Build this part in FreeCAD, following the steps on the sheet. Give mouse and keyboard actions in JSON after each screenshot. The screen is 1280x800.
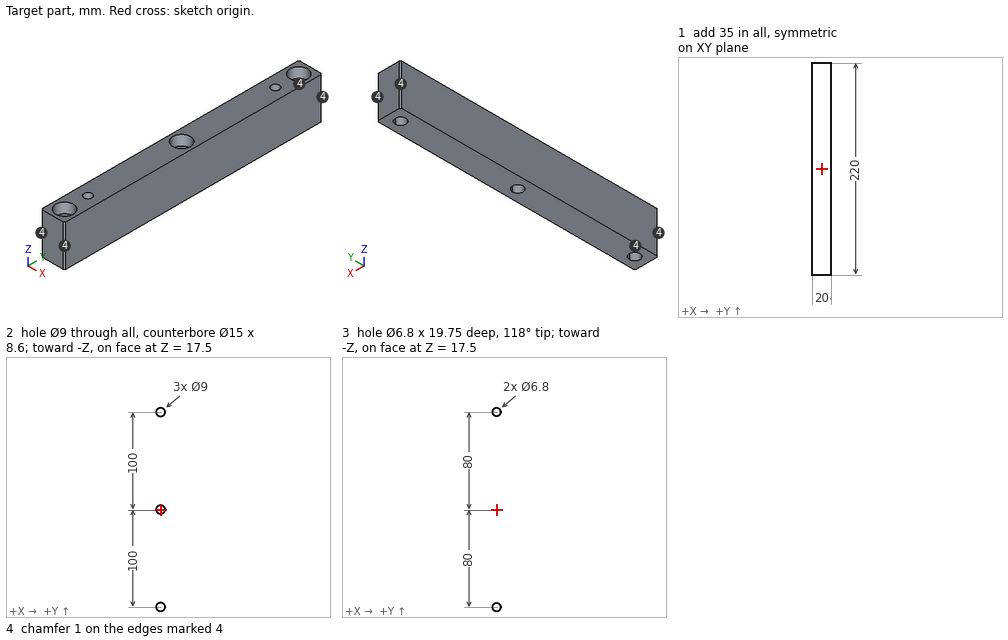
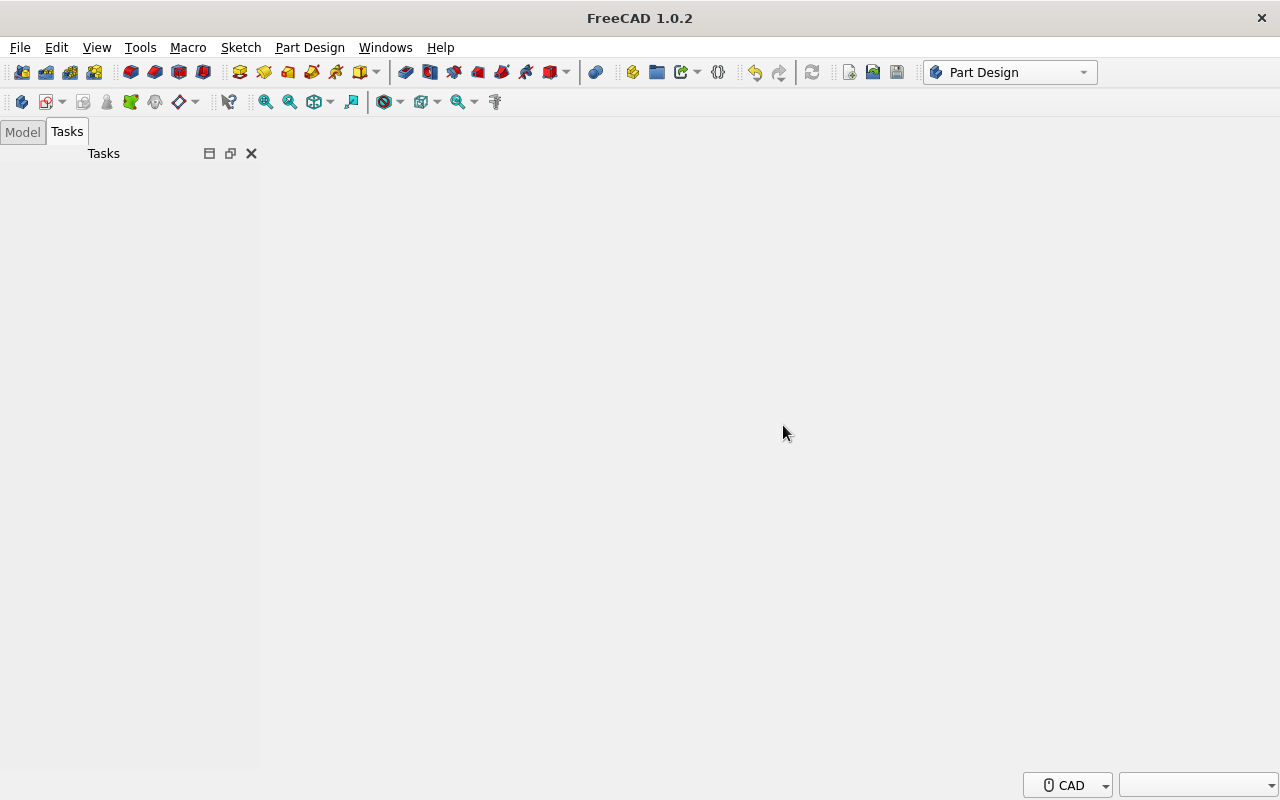
{"action": "left_click", "coordinate": [850, 72]}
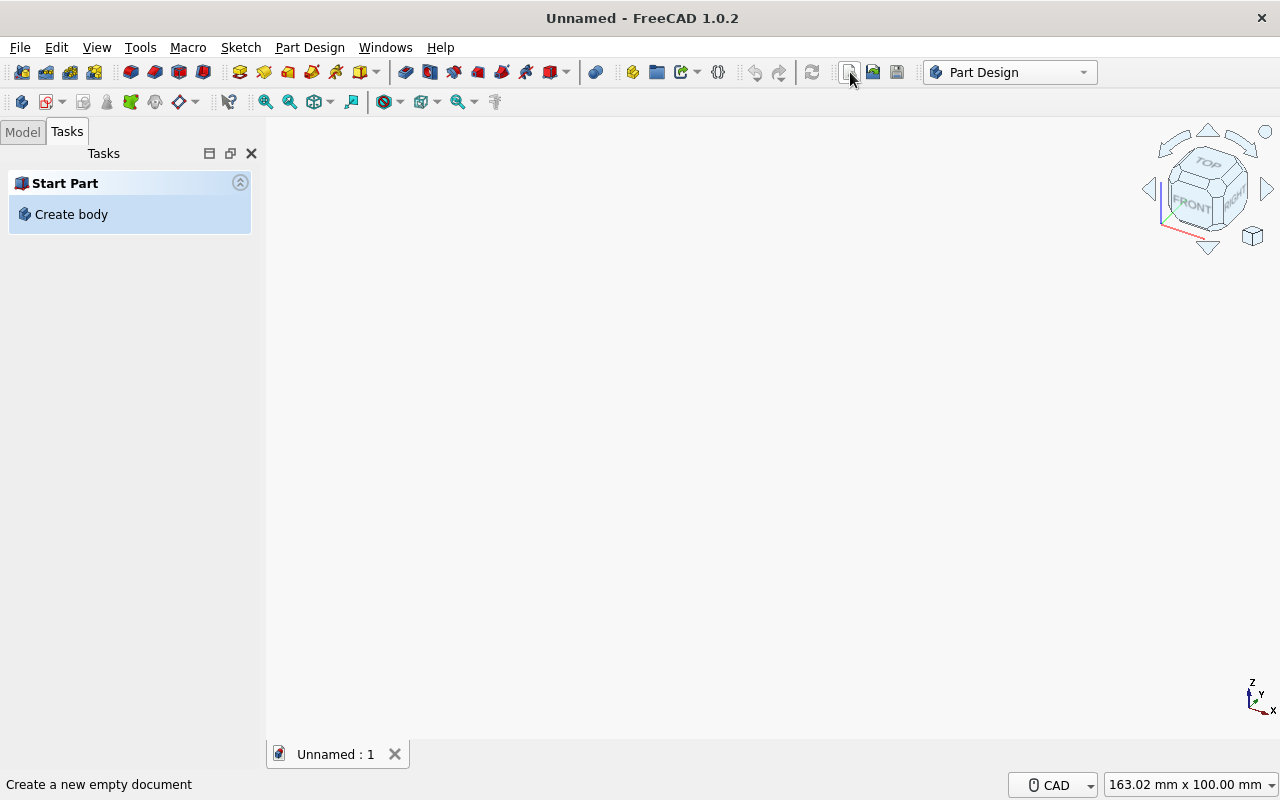
{"action": "left_click", "coordinate": [46, 102]}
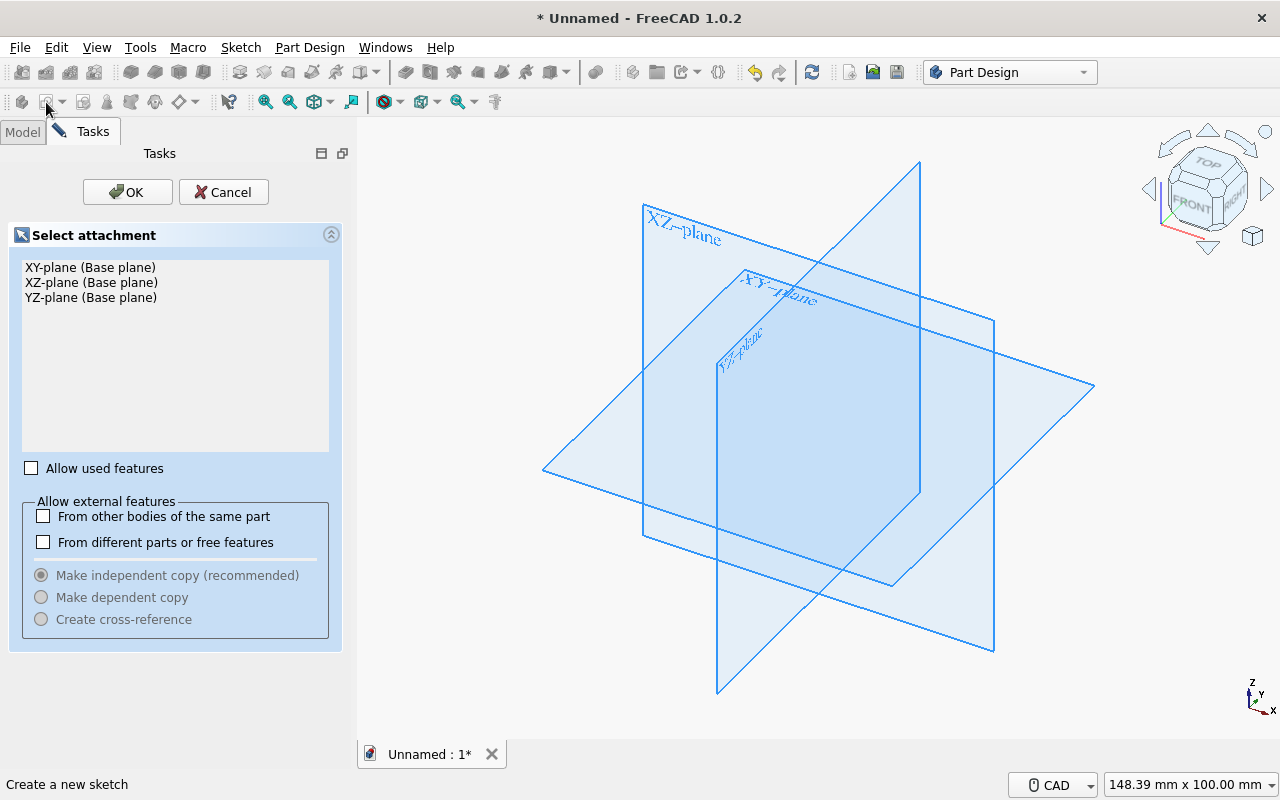
{"action": "left_click", "coordinate": [82, 268]}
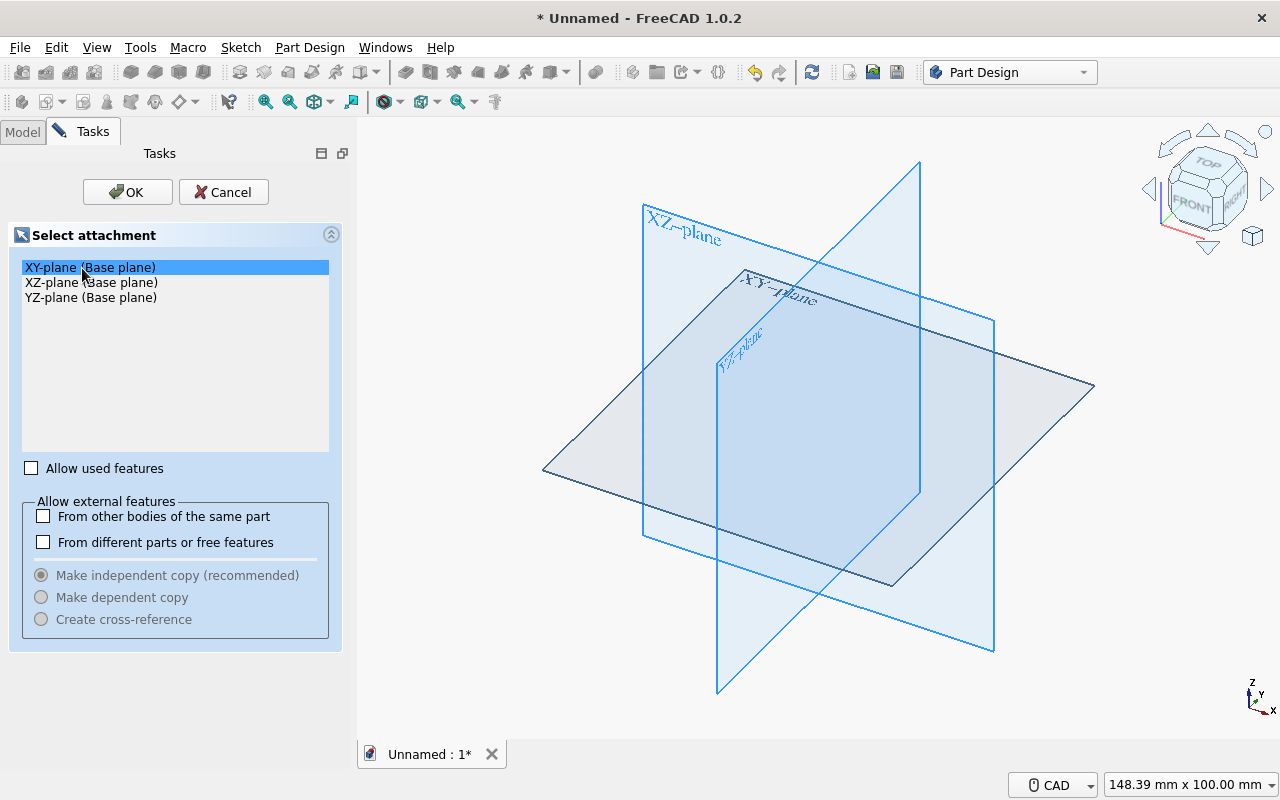
{"action": "left_click", "coordinate": [128, 192]}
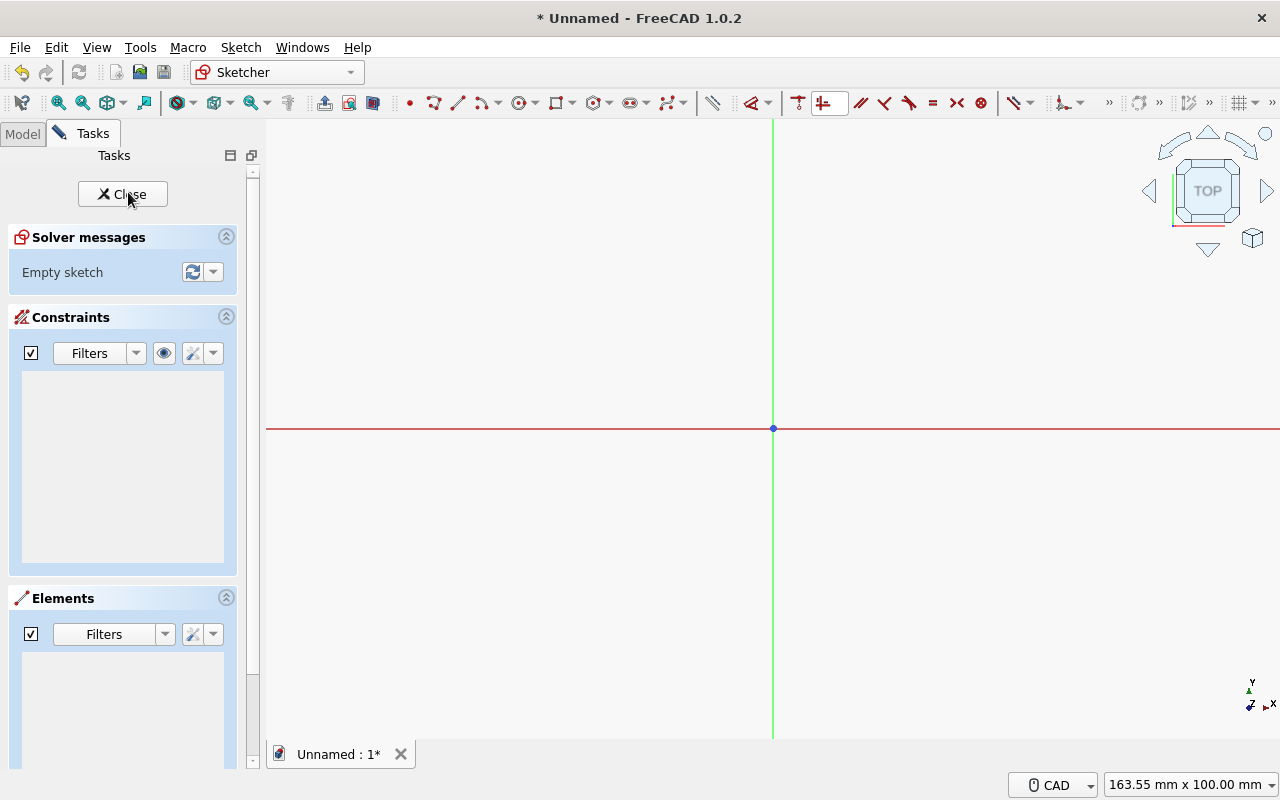
{"action": "scroll", "coordinate": [675, 429], "scroll_direction": "down", "scroll_amount": 6}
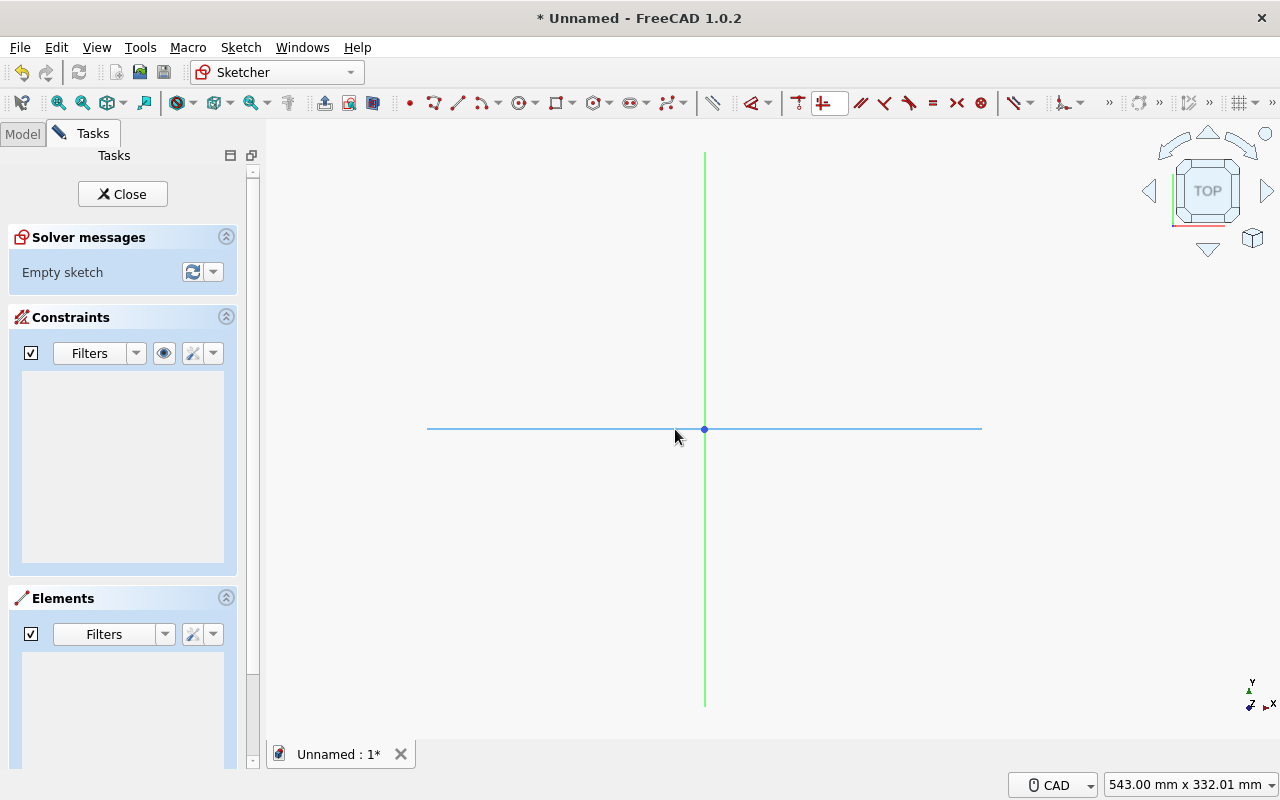
{"action": "left_click", "coordinate": [574, 104]}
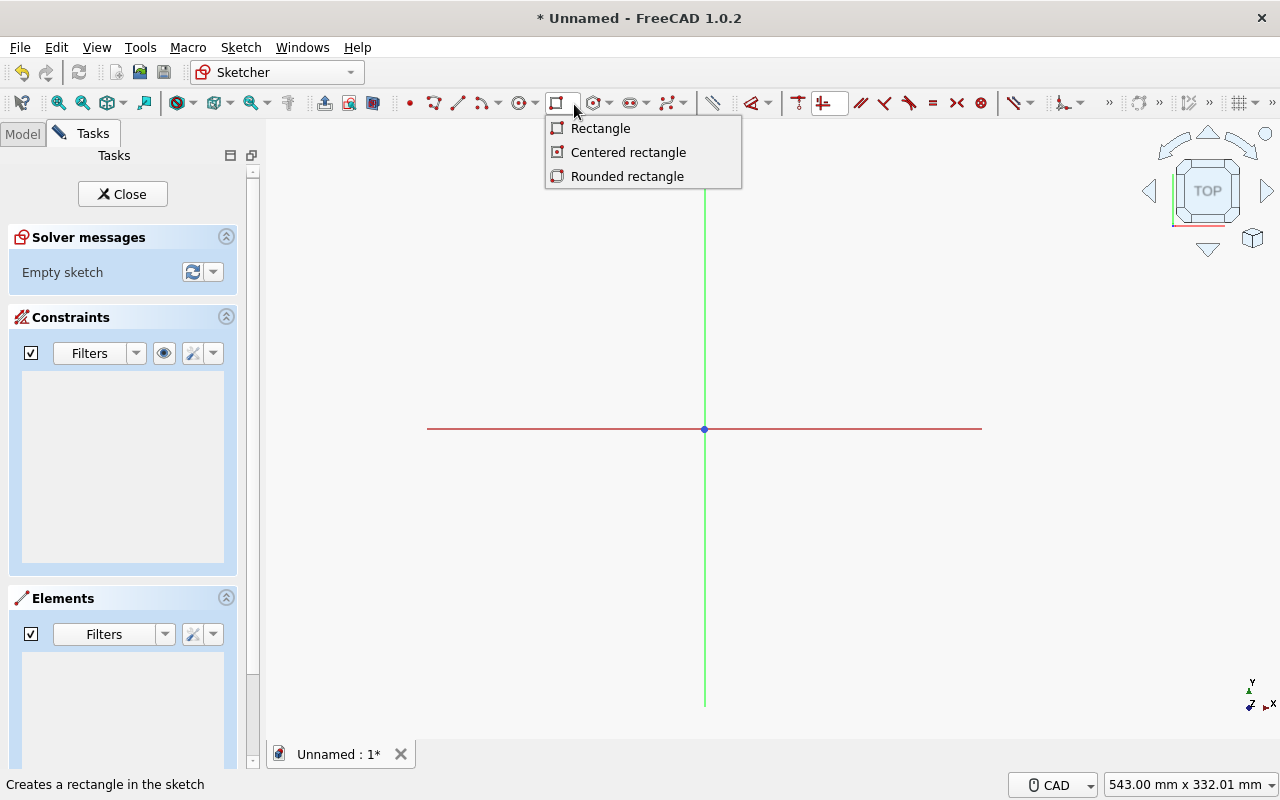
{"action": "left_click", "coordinate": [644, 152]}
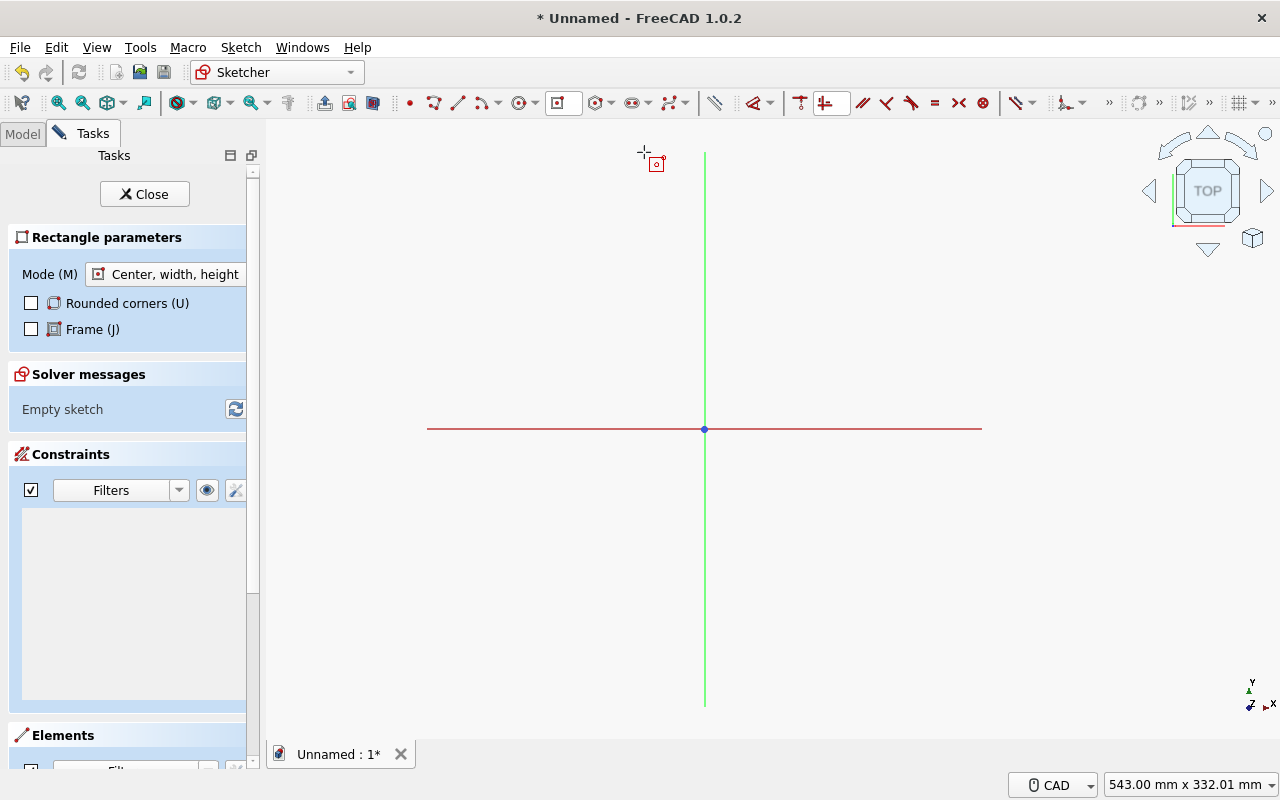
{"action": "left_click", "coordinate": [705, 429]}
{"action": "left_click", "coordinate": [723, 224]}
{"action": "key", "text": "Escape"}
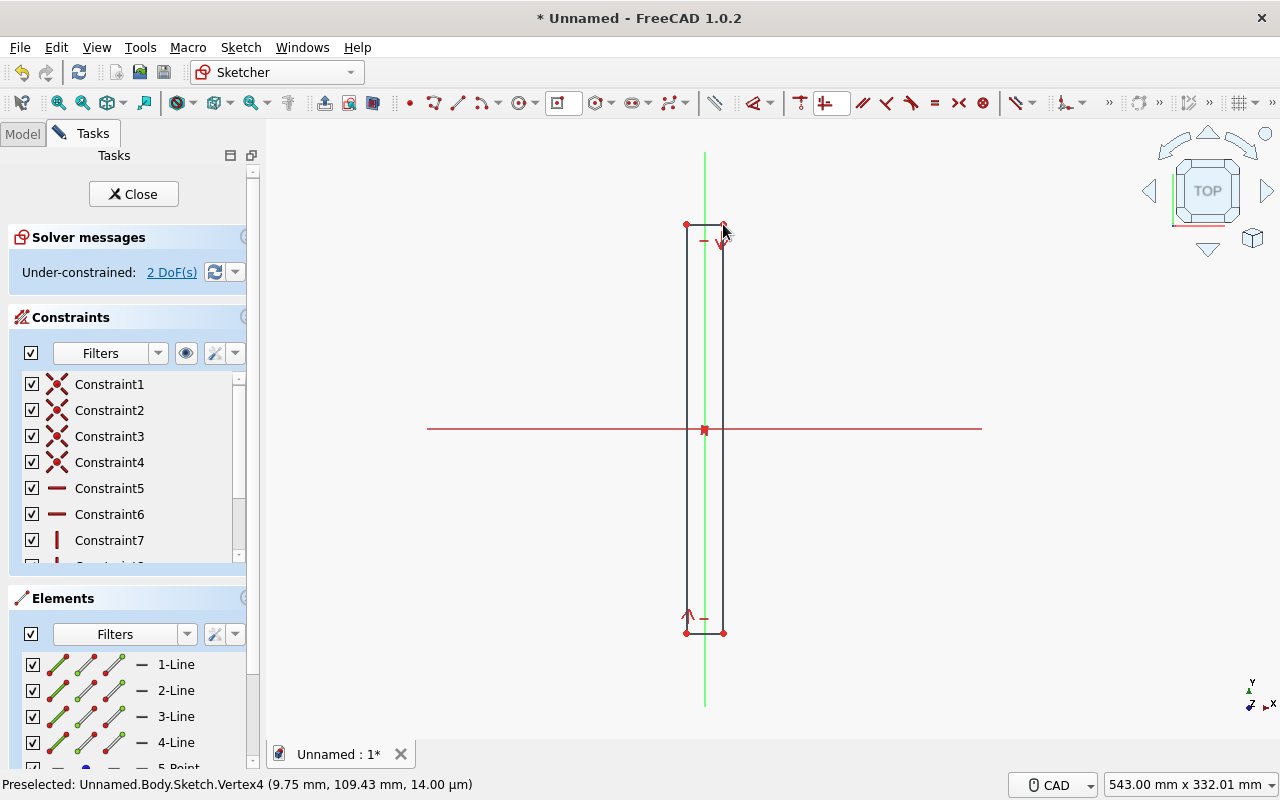
{"action": "left_click", "coordinate": [754, 104]}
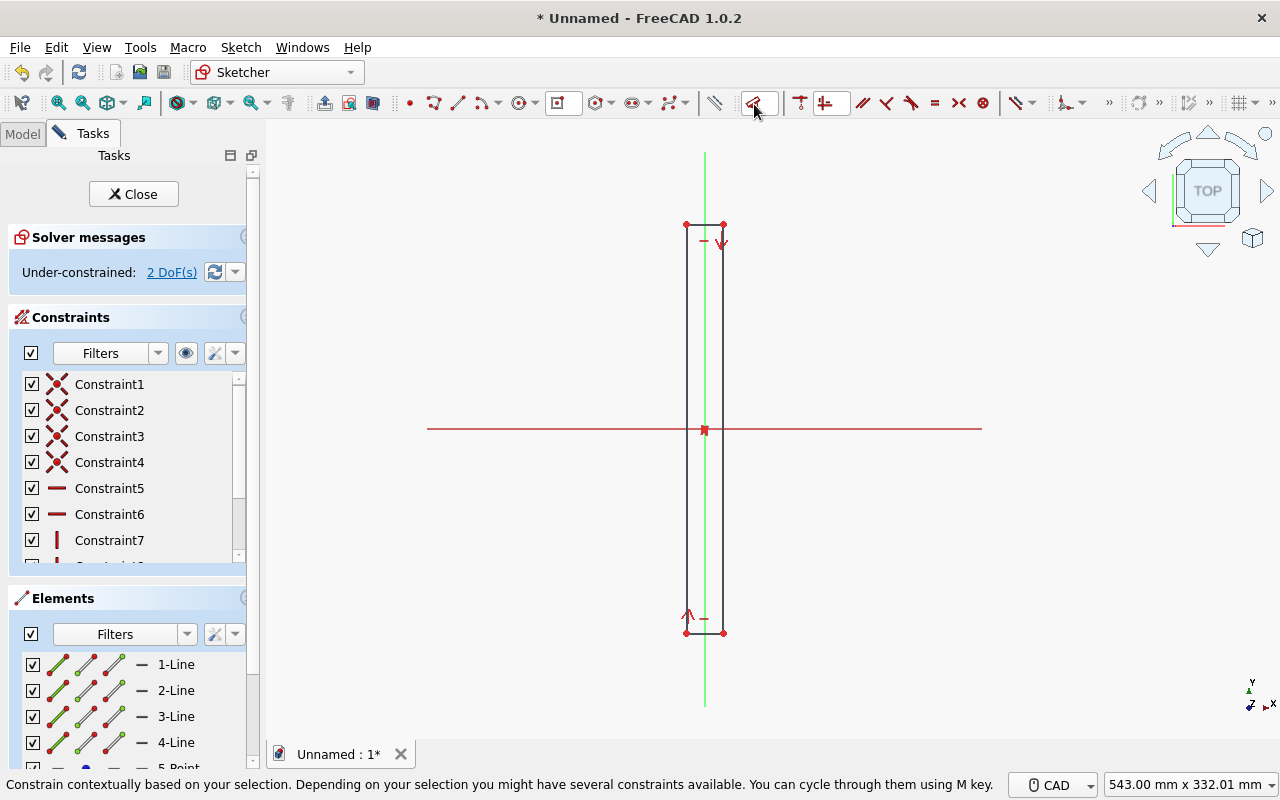
{"action": "left_click", "coordinate": [701, 634]}
{"action": "left_click", "coordinate": [696, 668]}